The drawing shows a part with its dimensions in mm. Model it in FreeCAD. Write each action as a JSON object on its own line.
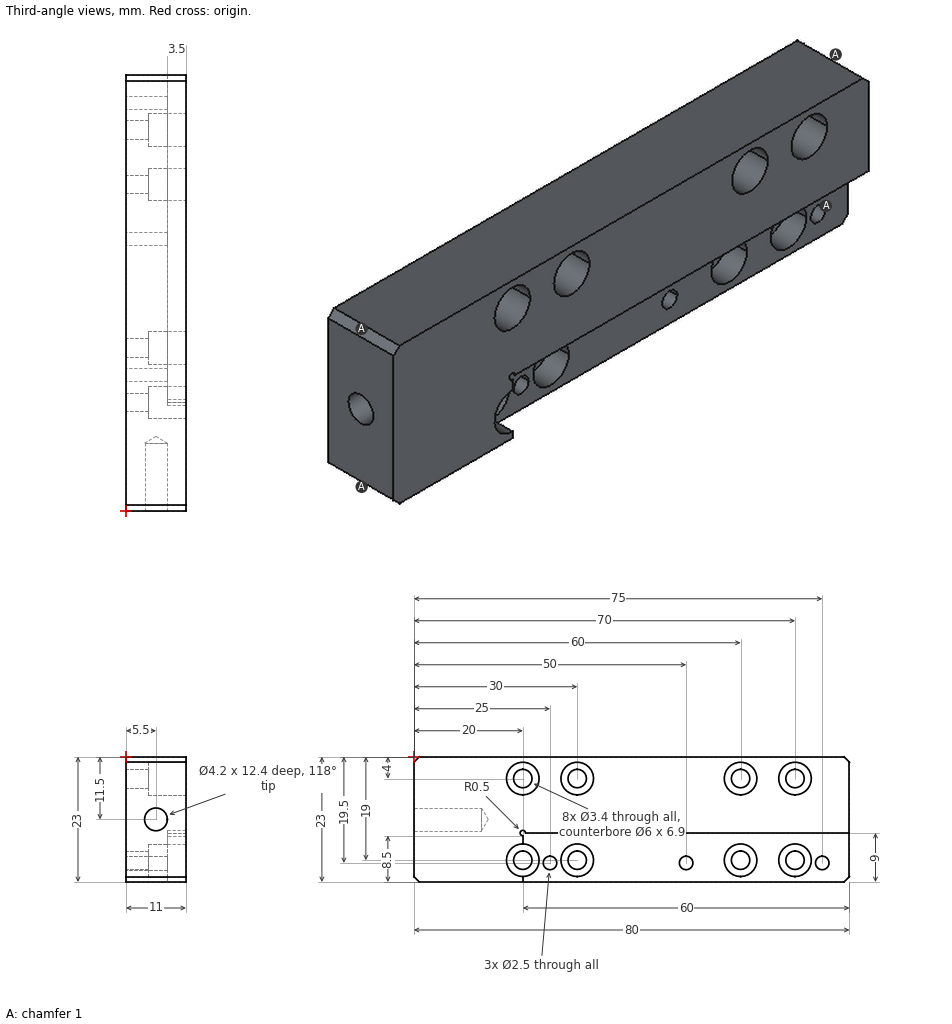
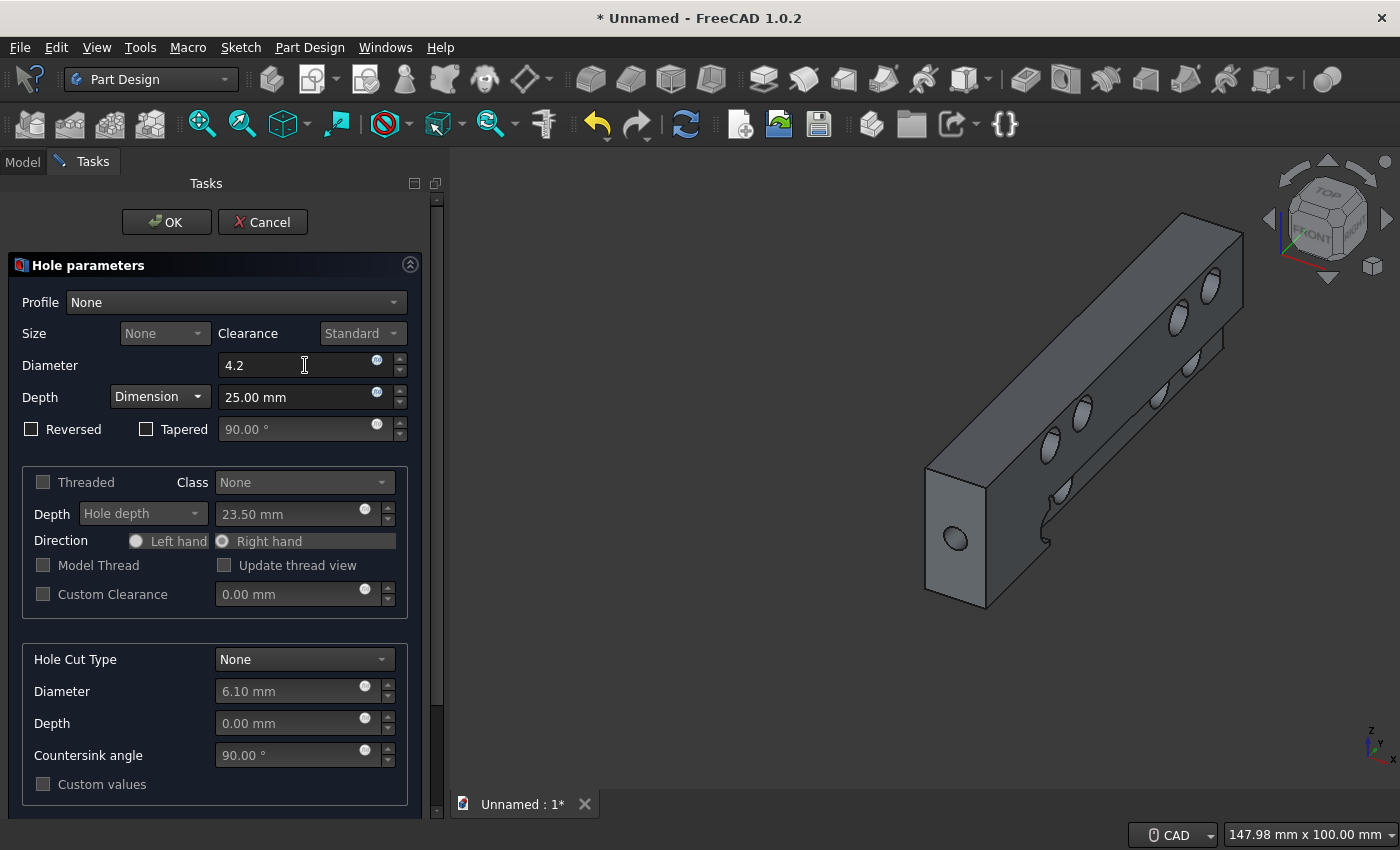
{"action": "triple_click", "coordinate": [305, 397]}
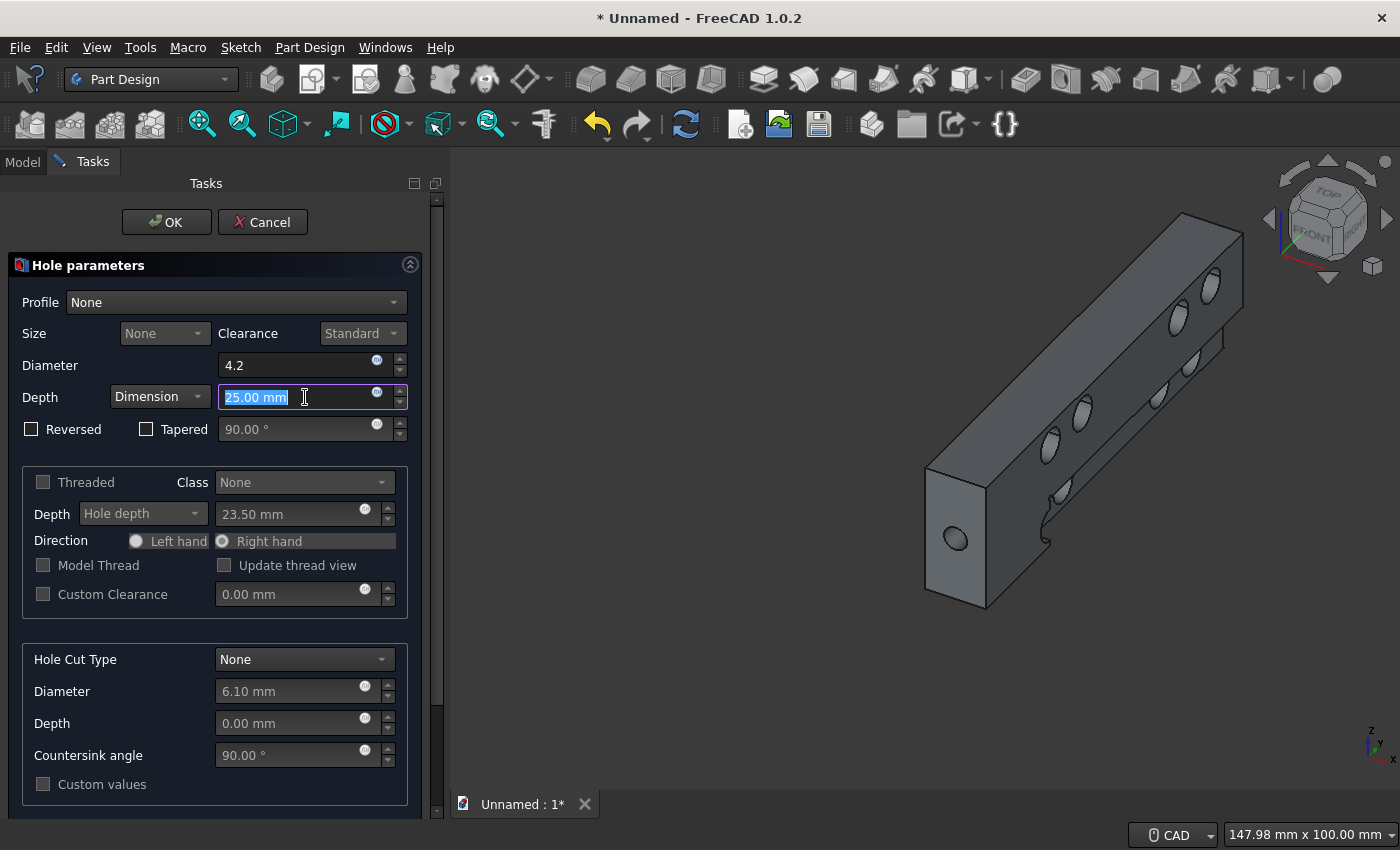
{"action": "type", "text": "12.4"}
{"action": "key", "text": "Tab"}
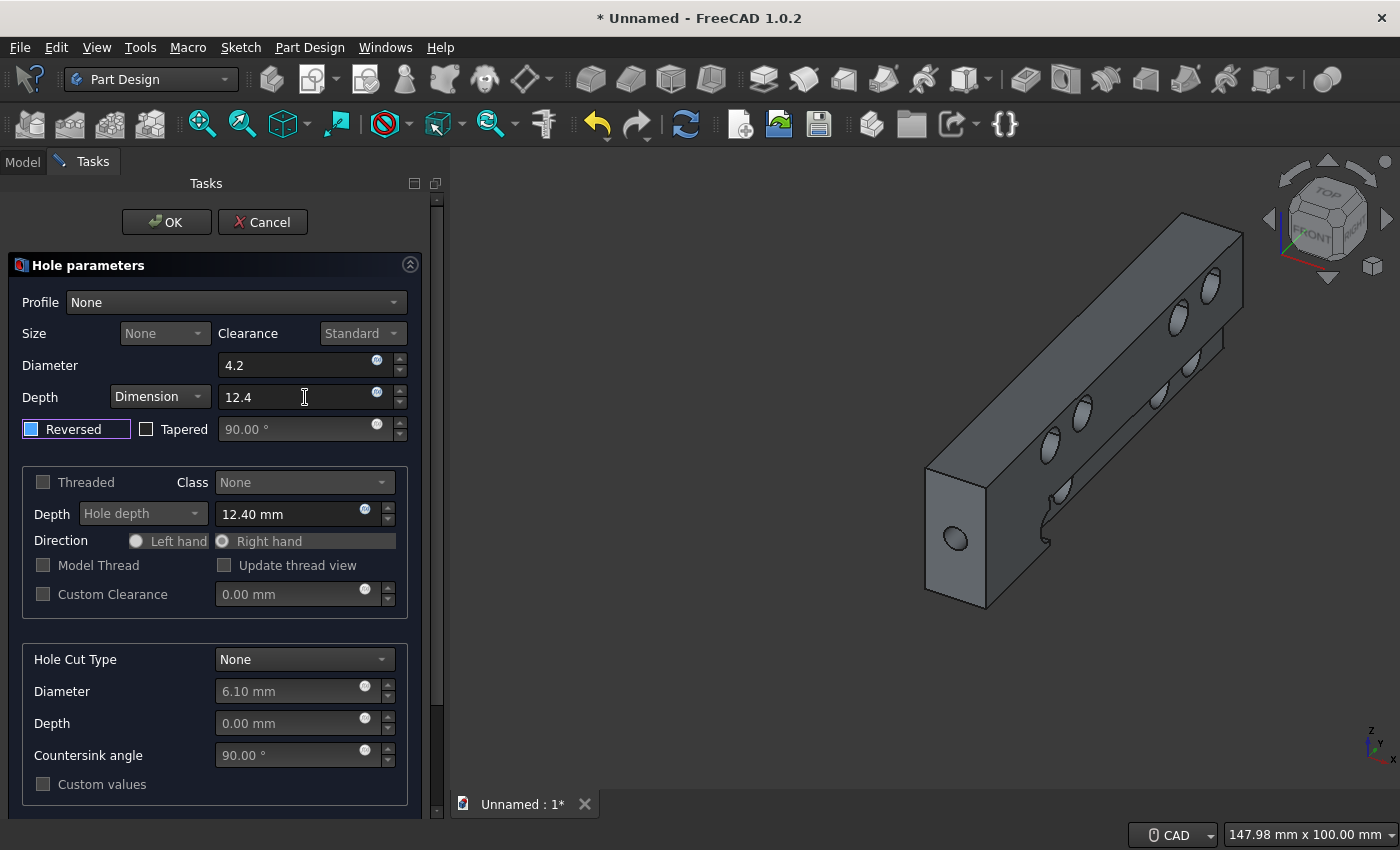
{"action": "left_click", "coordinate": [167, 222]}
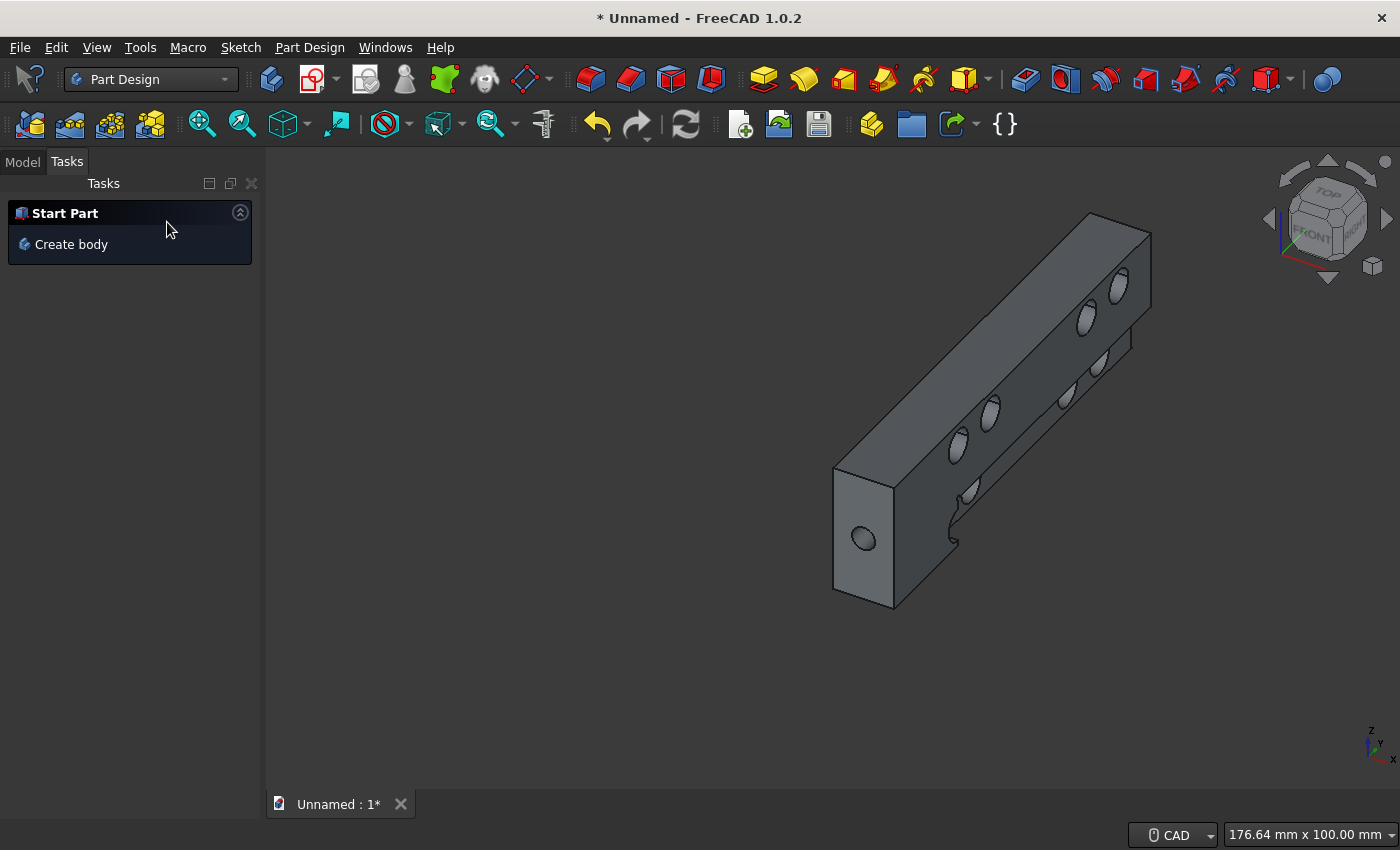
{"action": "key", "text": "0"}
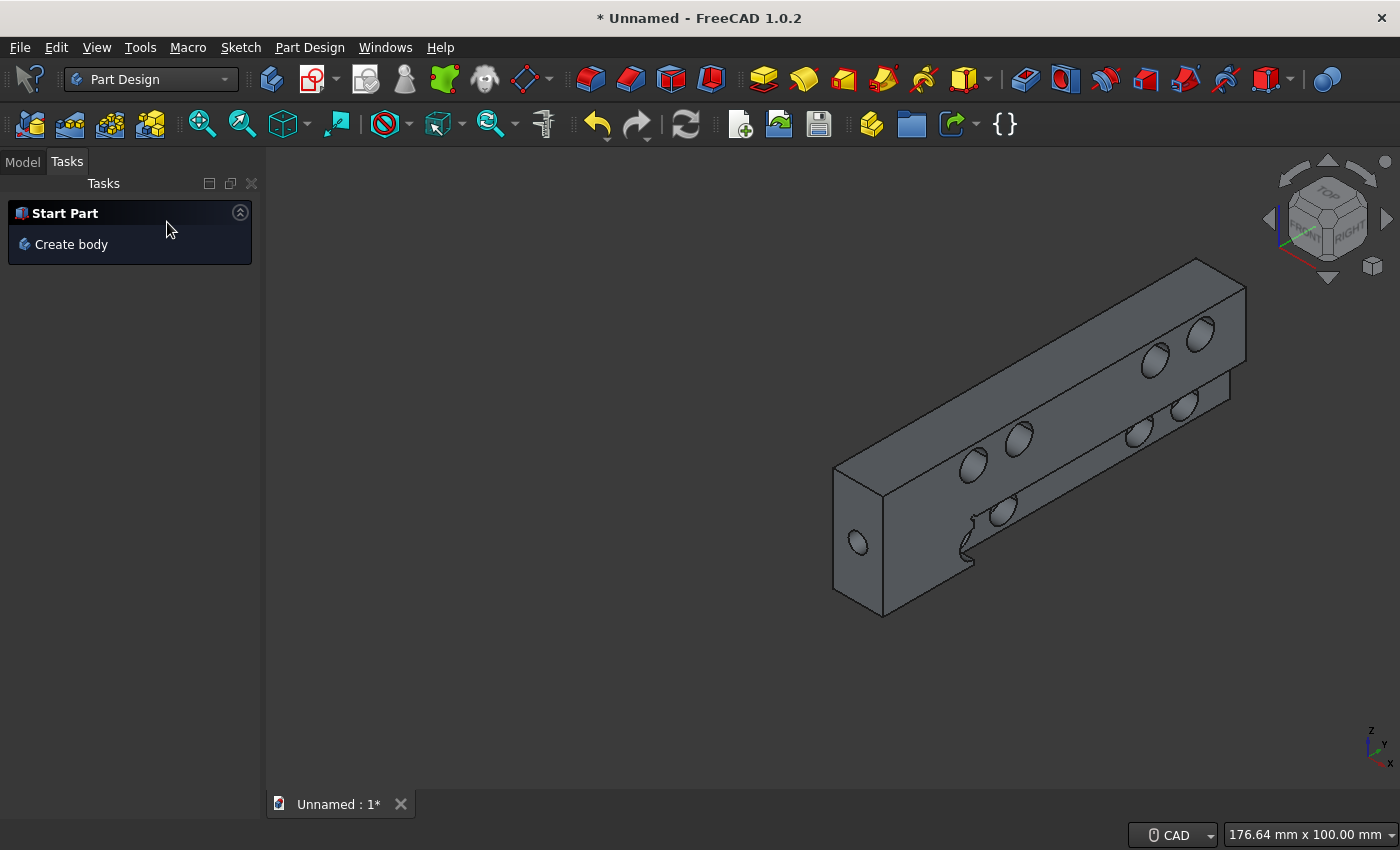
{"action": "left_click", "coordinate": [1093, 459]}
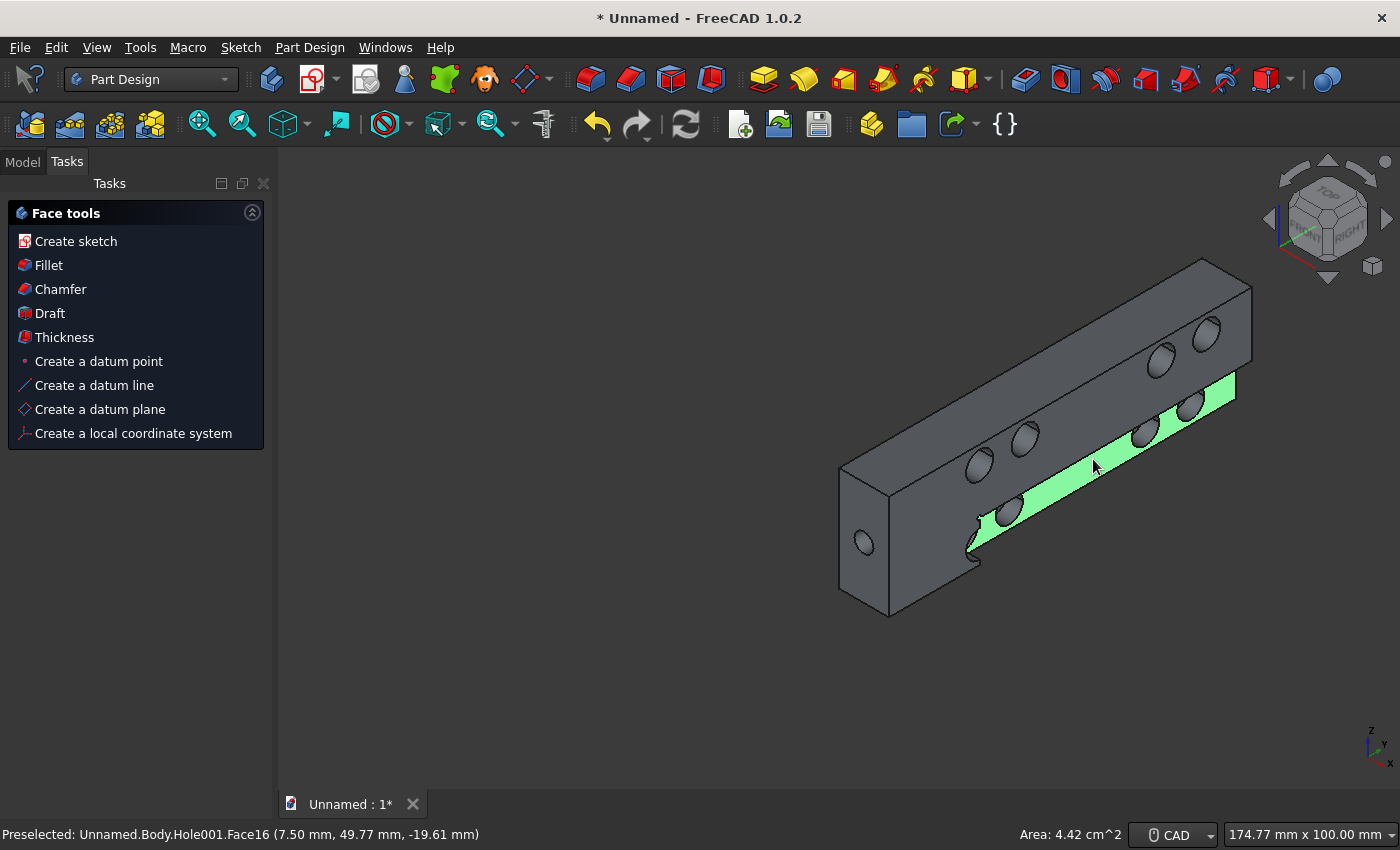
{"action": "left_click", "coordinate": [312, 80]}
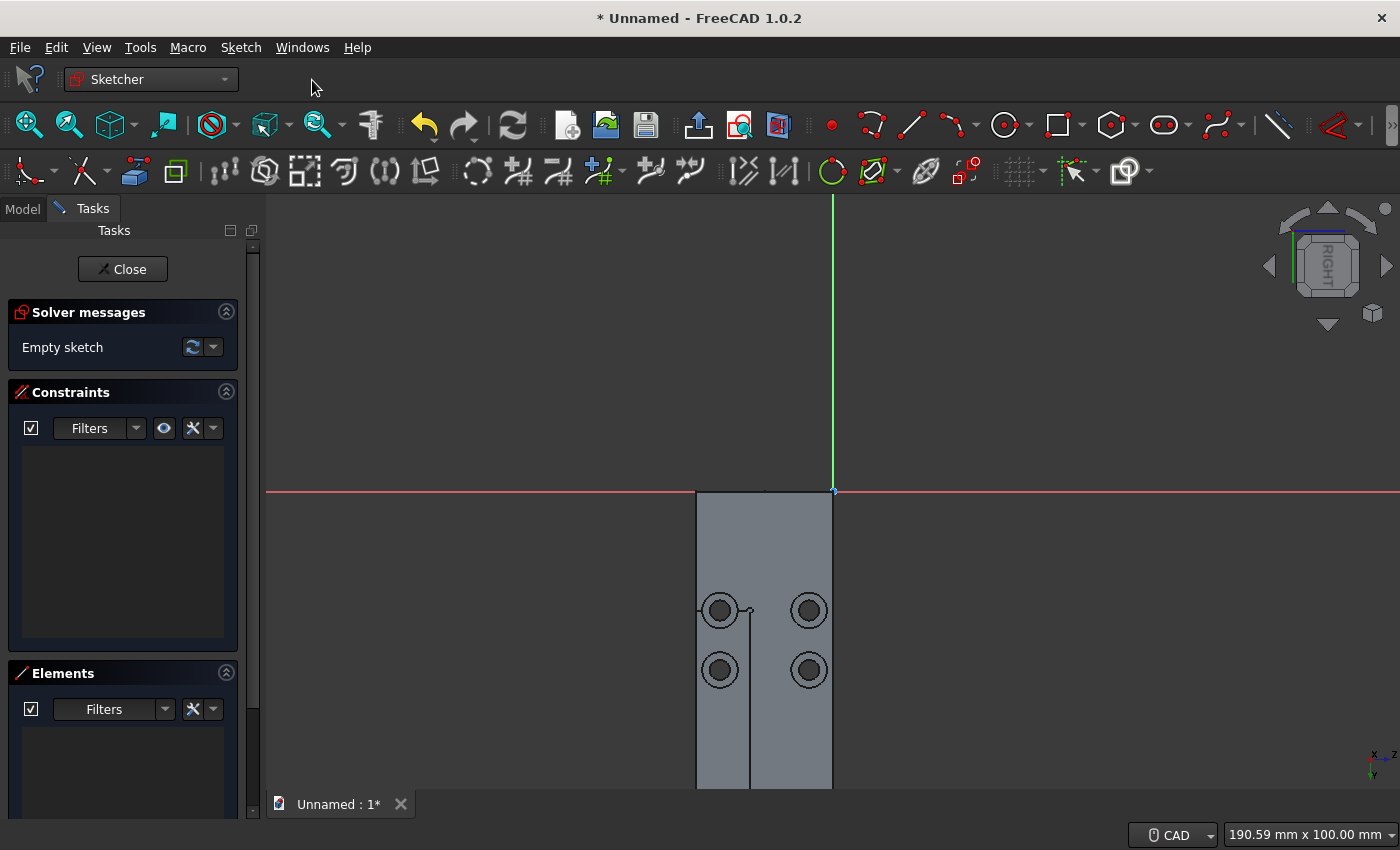
{"action": "scroll", "coordinate": [751, 222], "scroll_direction": "down", "scroll_amount": 2}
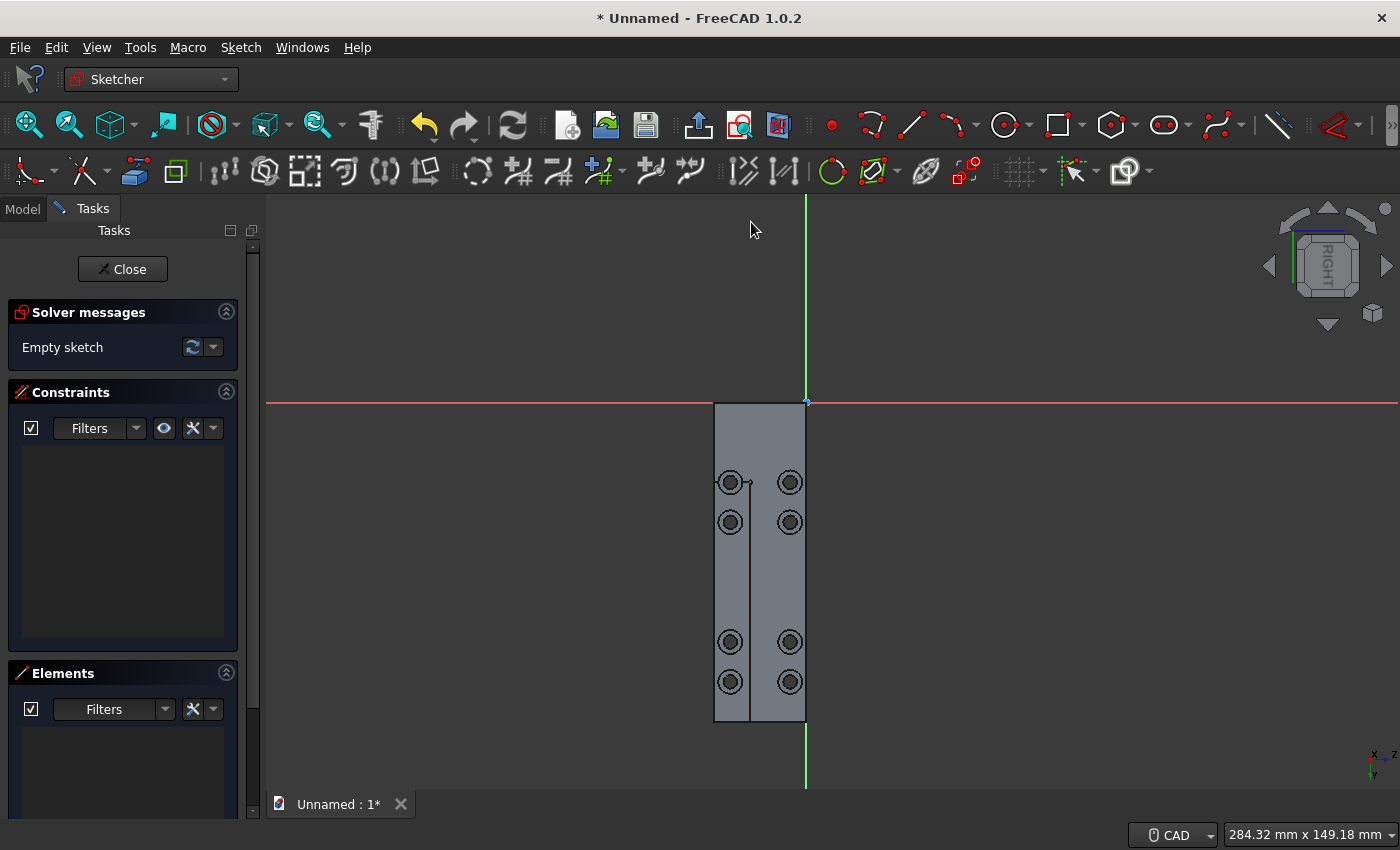
{"action": "left_click", "coordinate": [1006, 126]}